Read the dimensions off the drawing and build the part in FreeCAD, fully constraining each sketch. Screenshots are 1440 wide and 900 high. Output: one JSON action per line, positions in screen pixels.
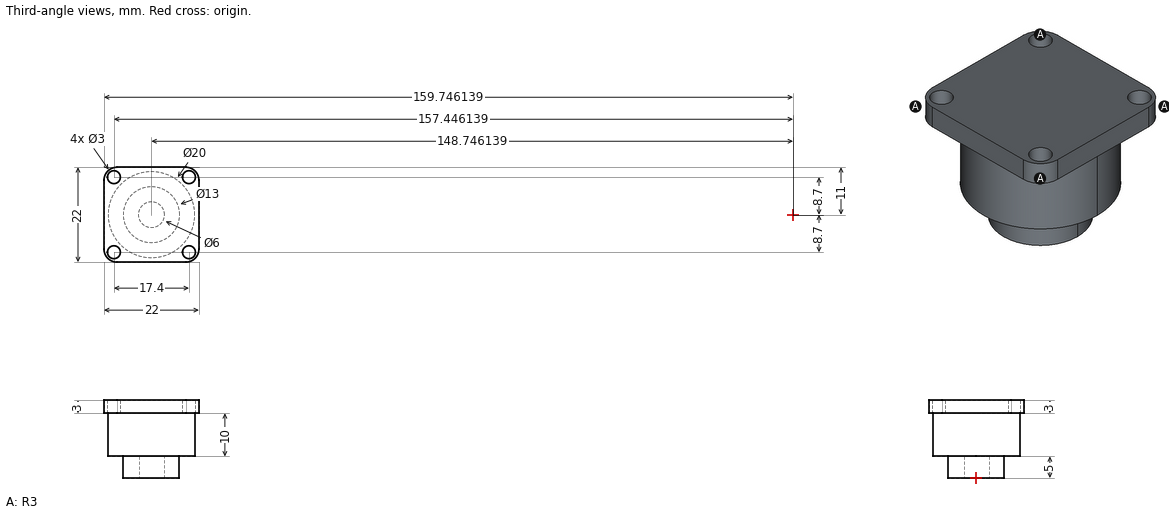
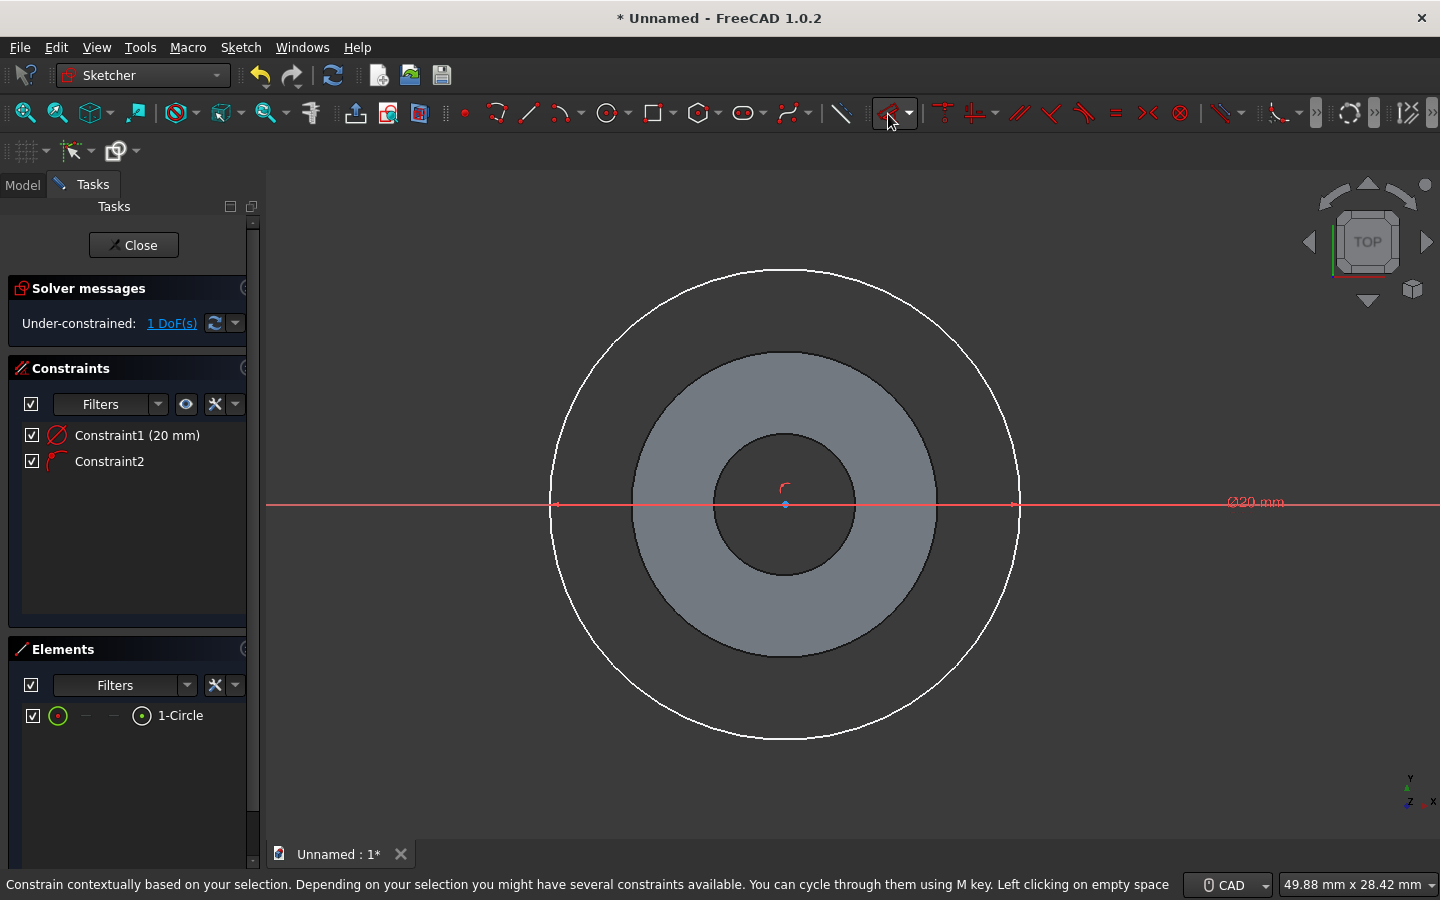
{"action": "left_click", "coordinate": [785, 504]}
{"action": "left_click", "coordinate": [917, 538]}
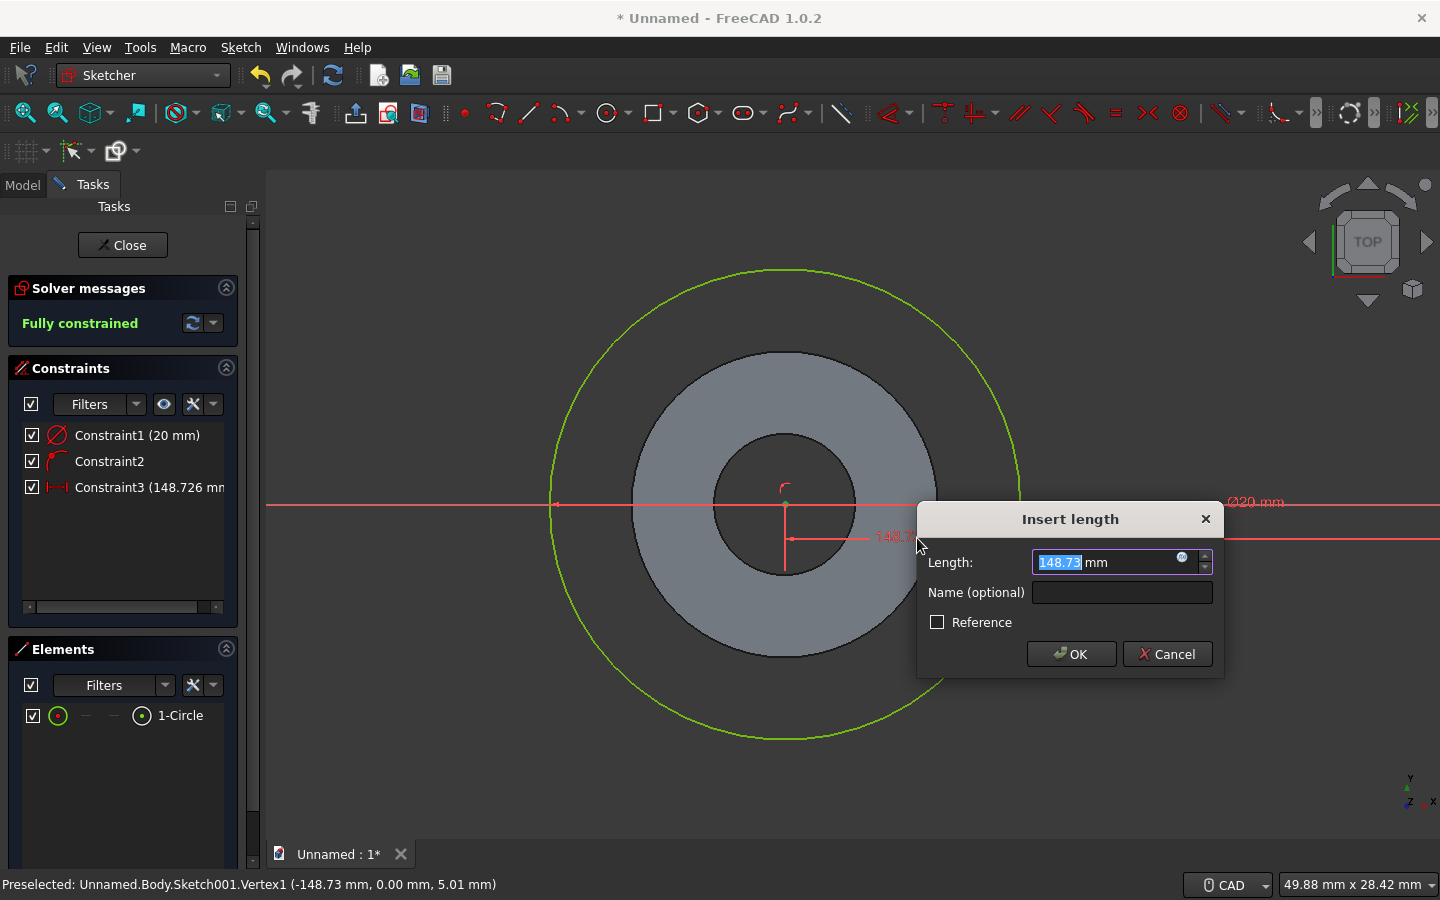
{"action": "type", "text": "148.746139"}
{"action": "key", "text": "Return"}
{"action": "key", "text": "Escape"}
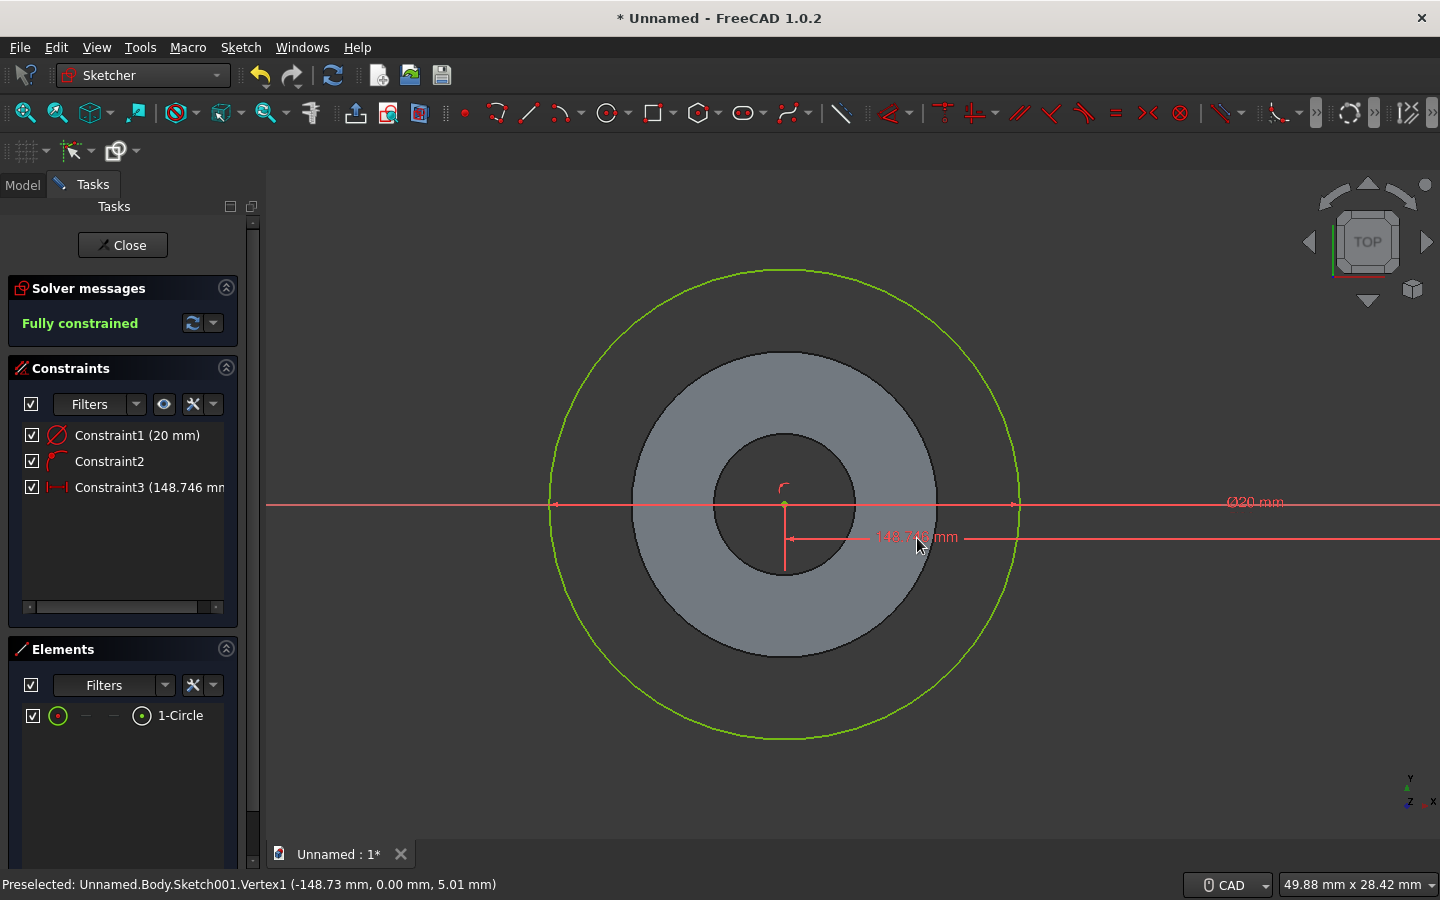
{"action": "left_click", "coordinate": [123, 245]}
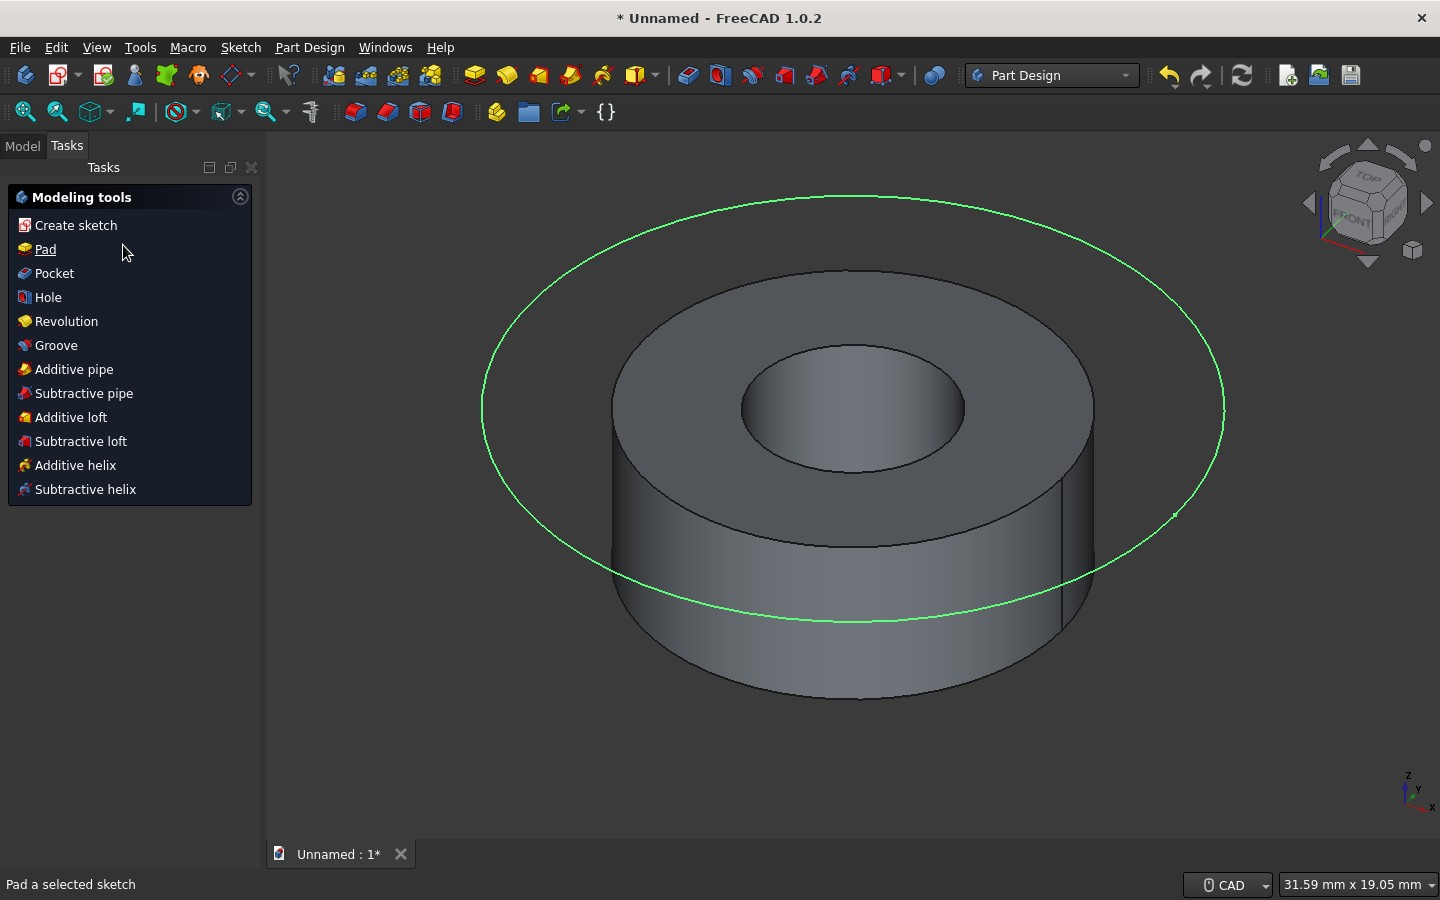
{"action": "left_click", "coordinate": [476, 76]}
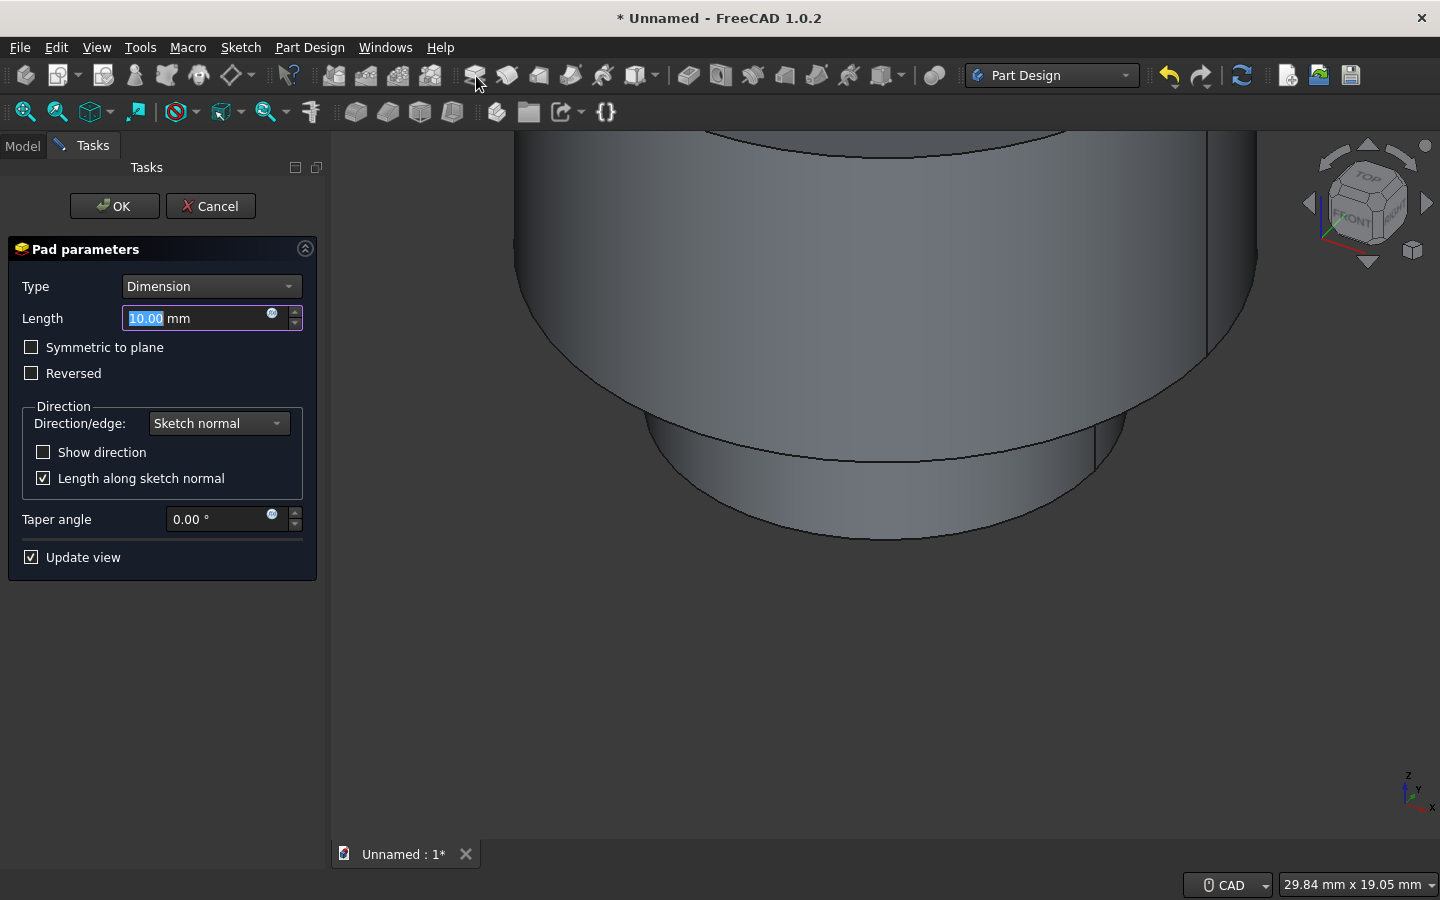
{"action": "type", "text": "10"}
{"action": "key", "text": "Tab"}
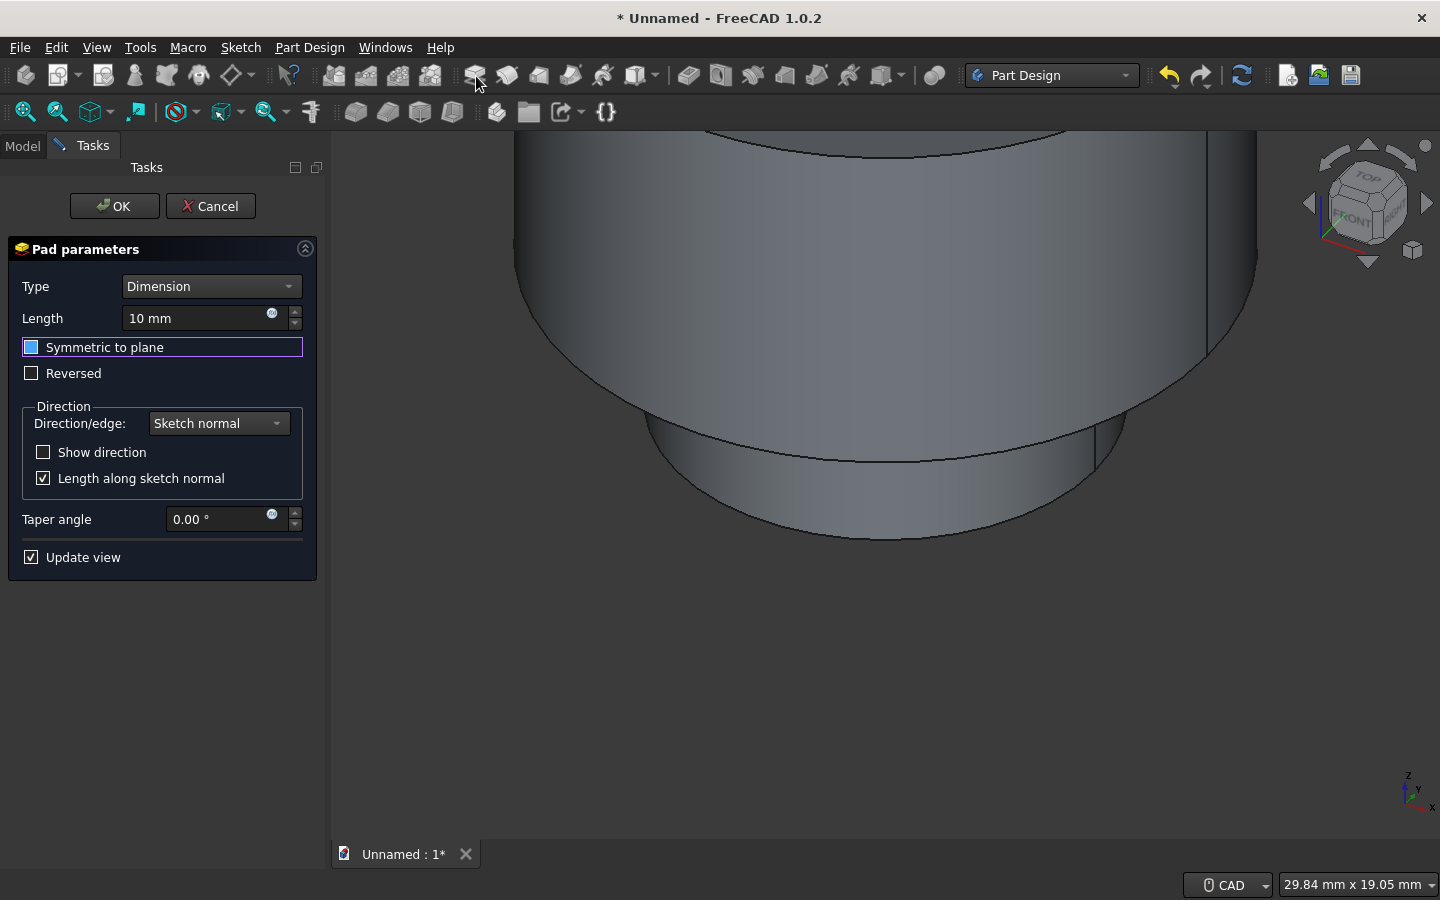
{"action": "left_click", "coordinate": [115, 206]}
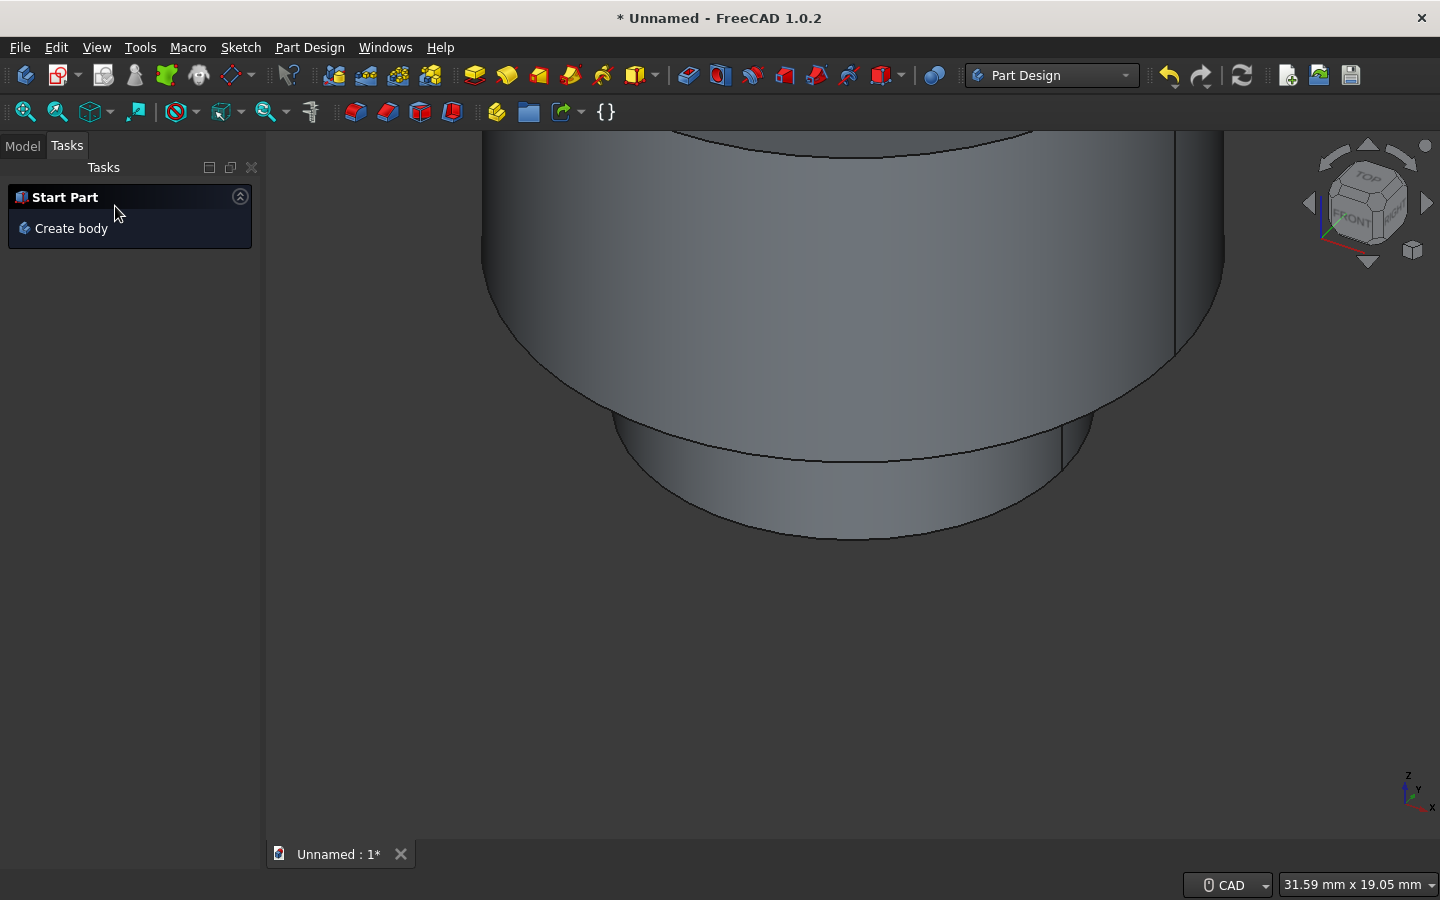
{"action": "left_click", "coordinate": [26, 112]}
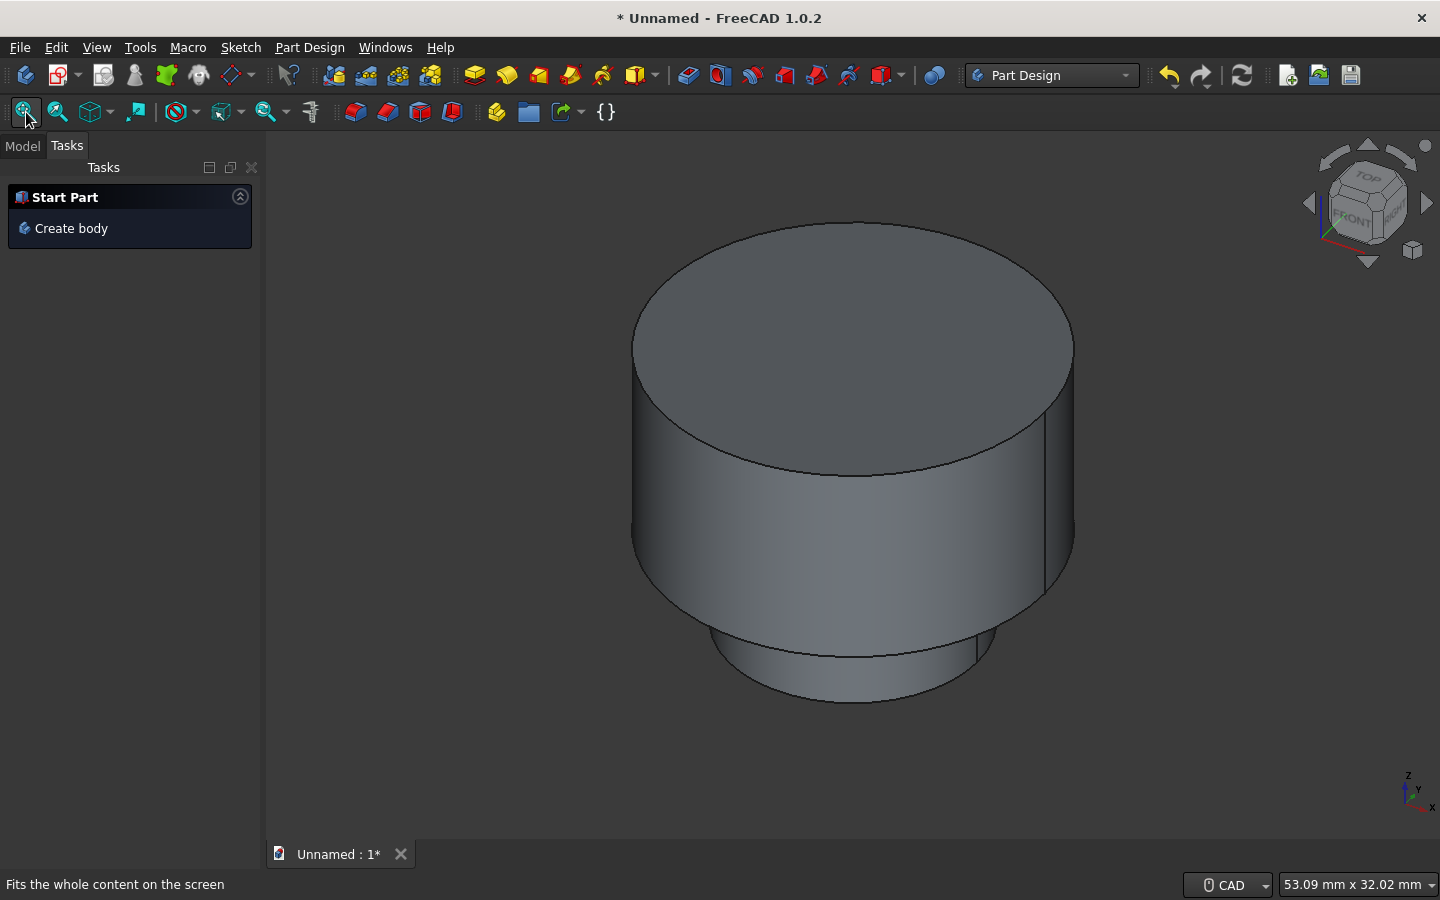
{"action": "left_click", "coordinate": [853, 348]}